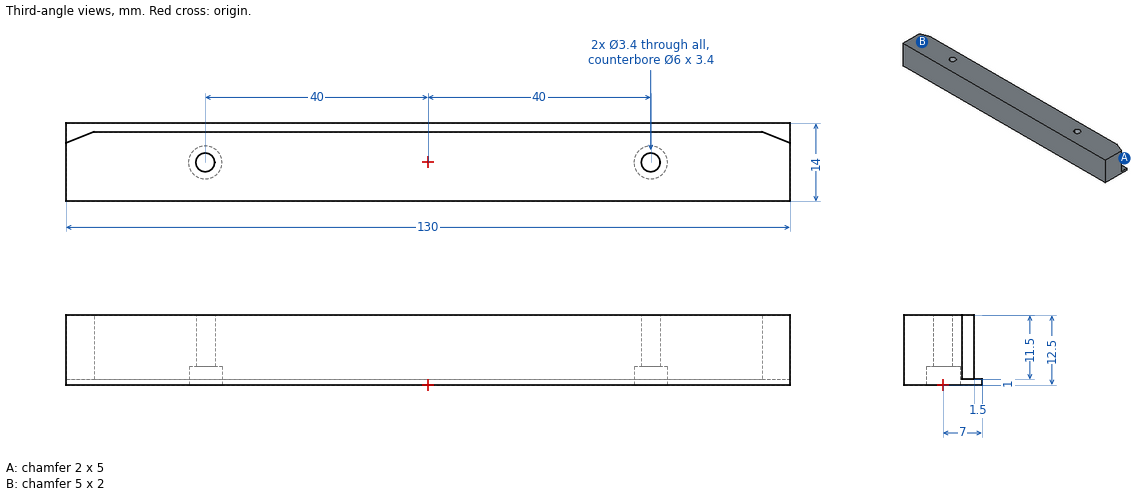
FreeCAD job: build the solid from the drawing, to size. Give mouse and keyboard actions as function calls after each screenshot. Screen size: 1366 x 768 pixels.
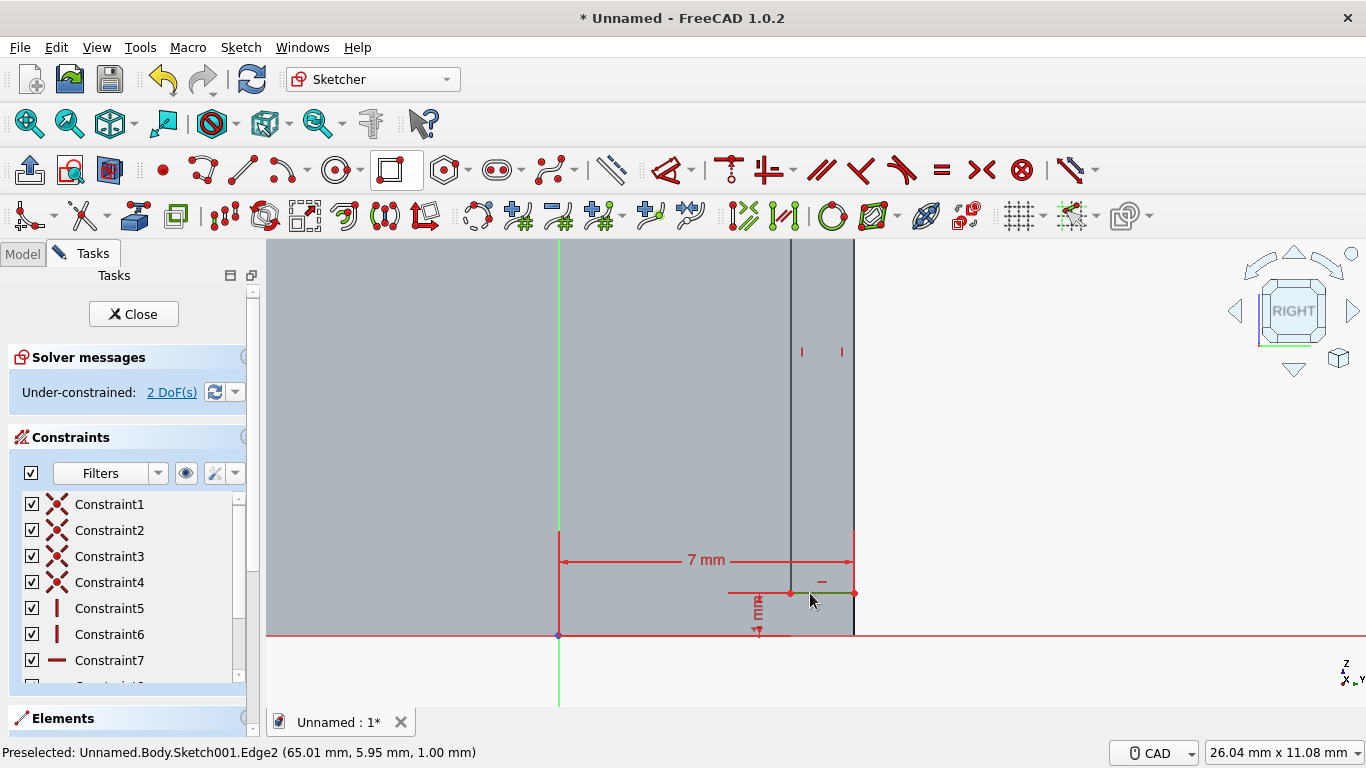
key(l)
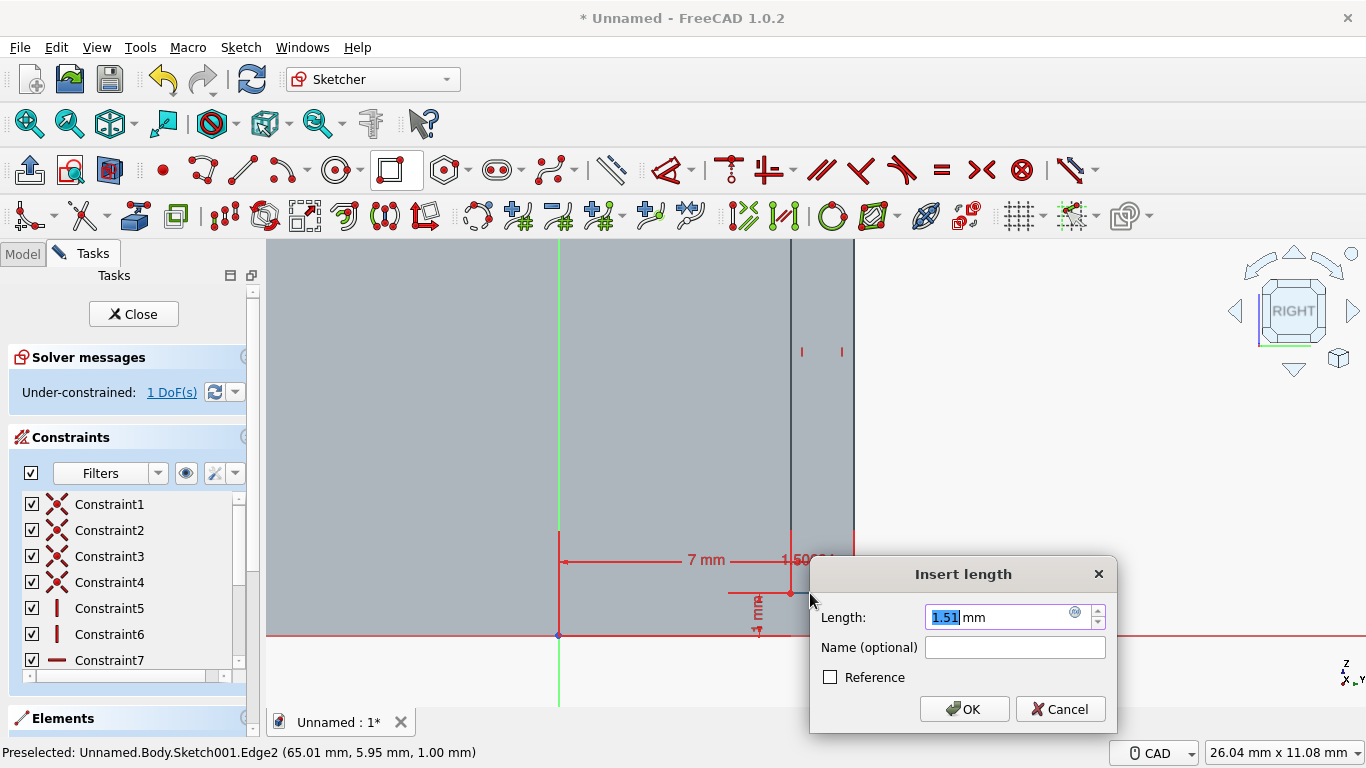
text(1.5)
key(Return)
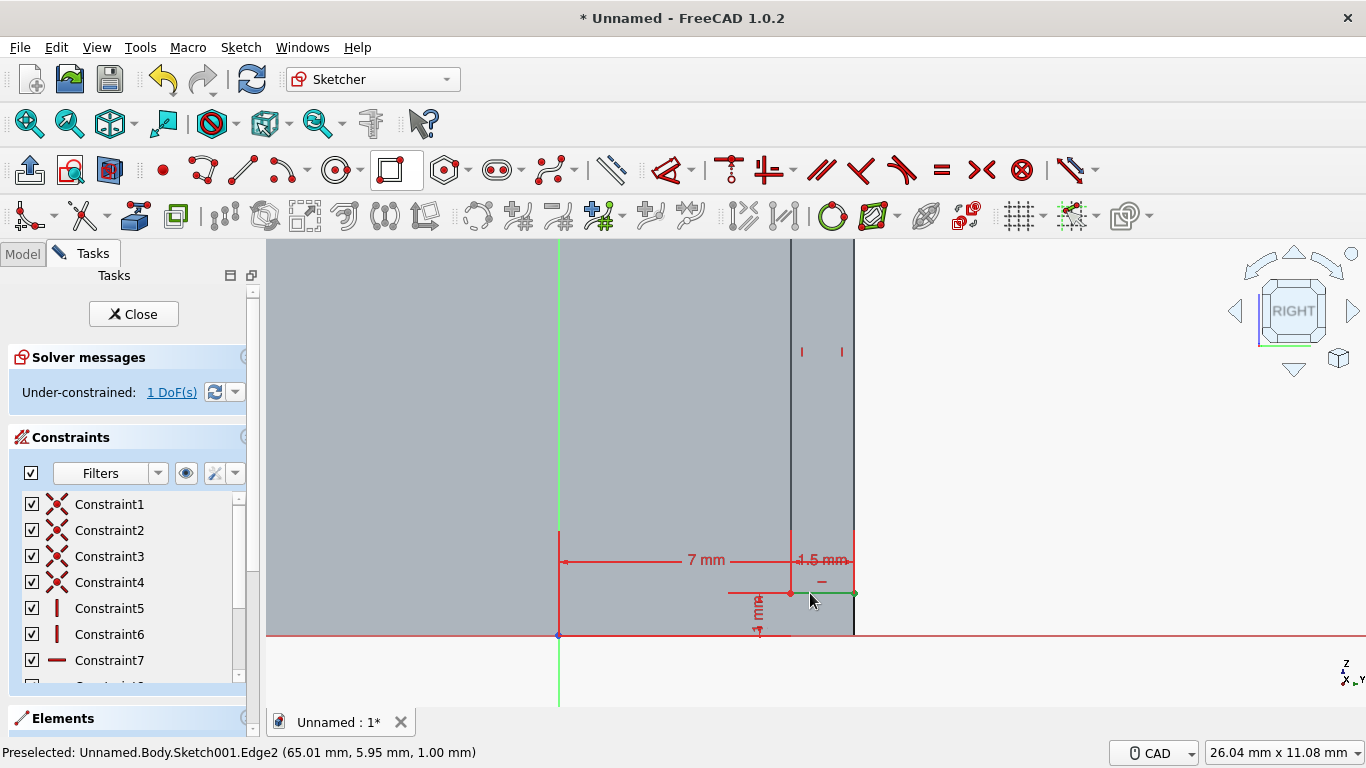
click(791, 448)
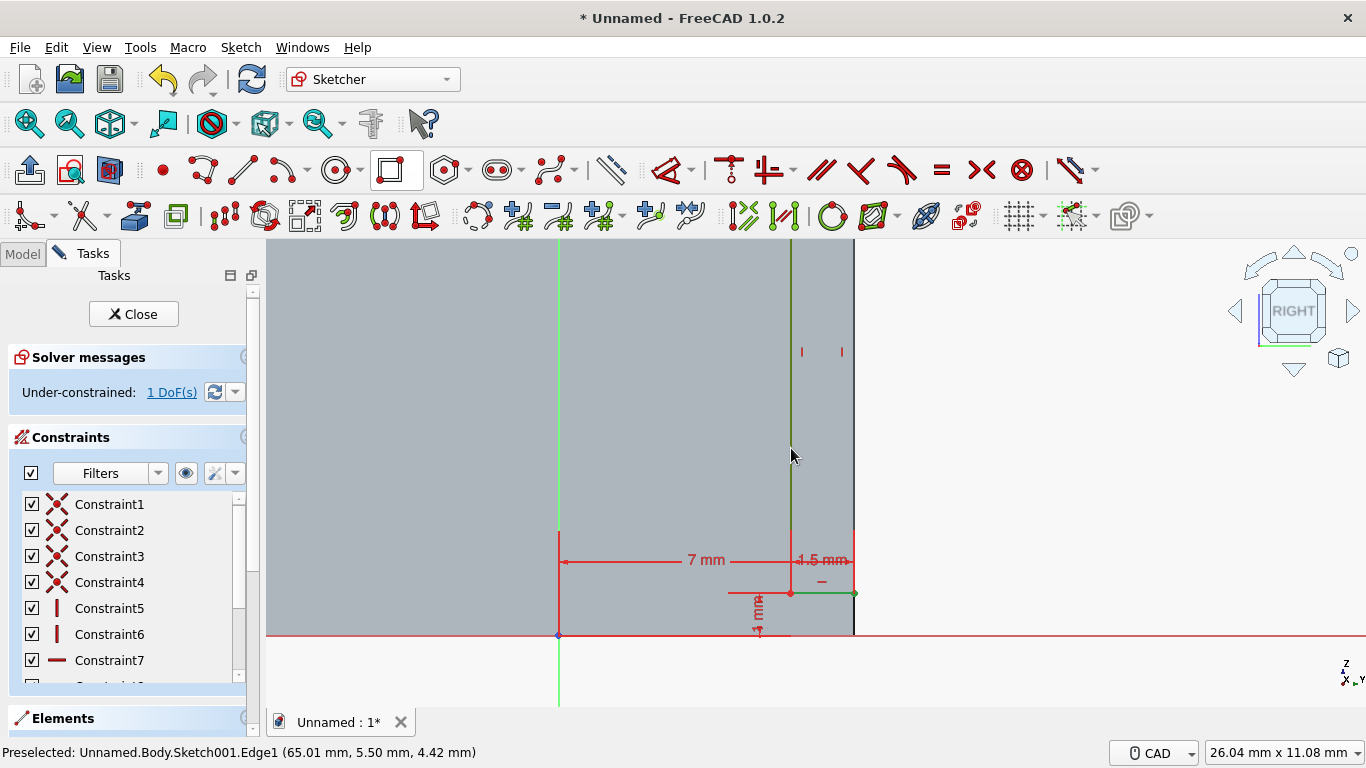
click(694, 170)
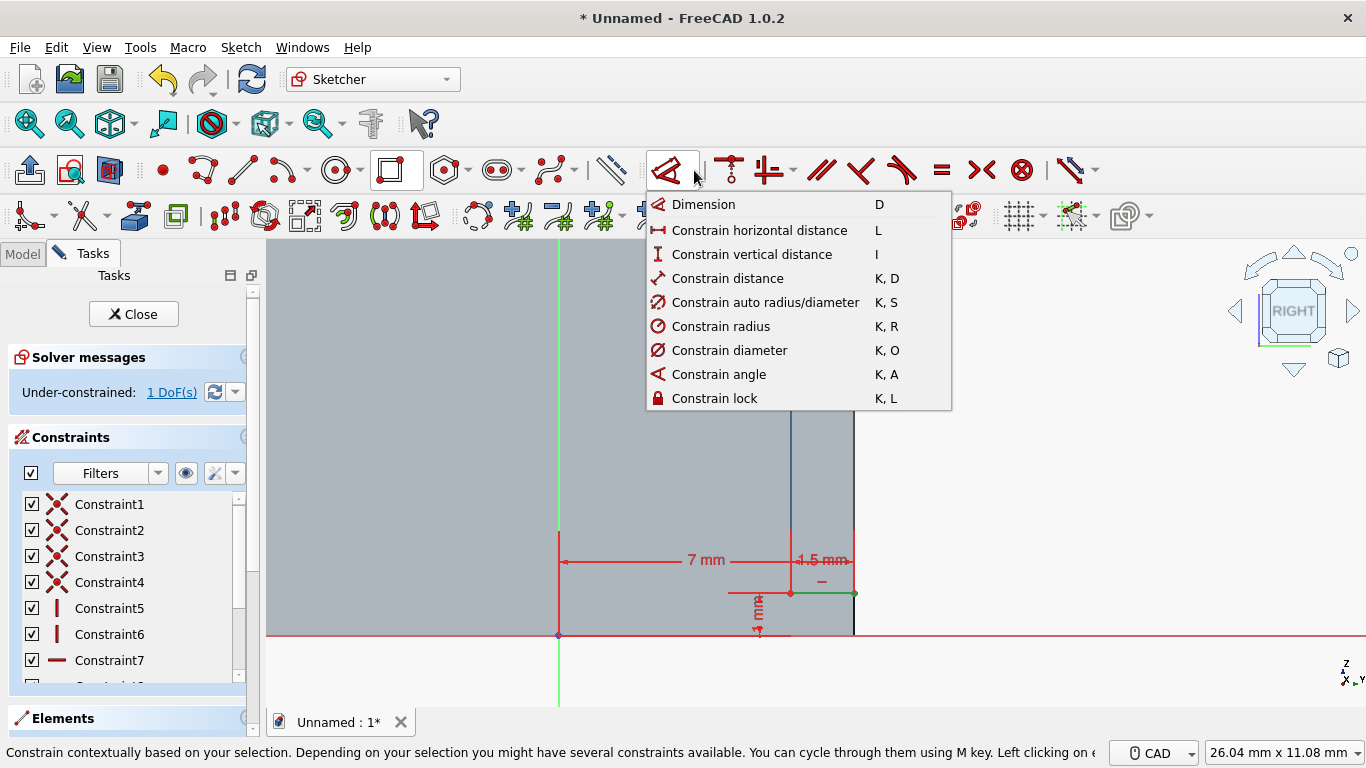
click(799, 254)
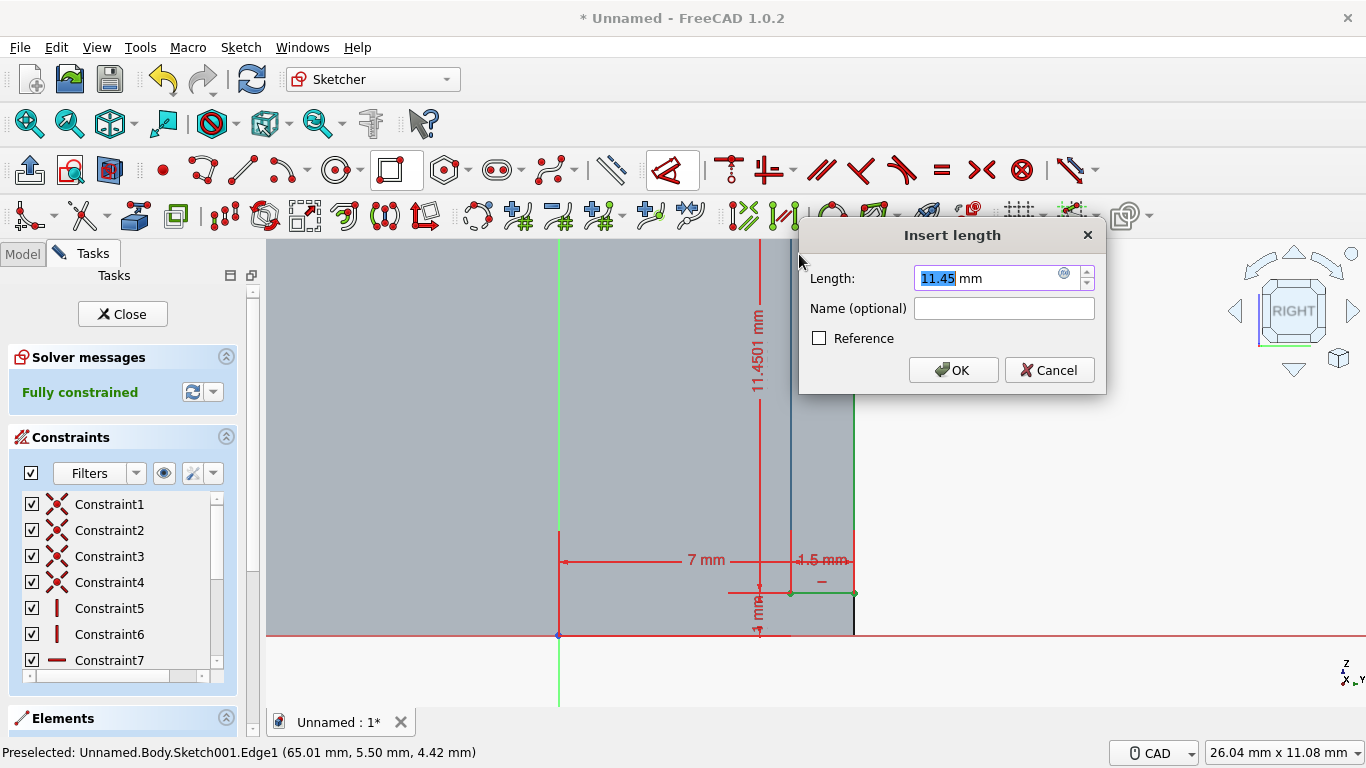
text(11.5)
key(Return)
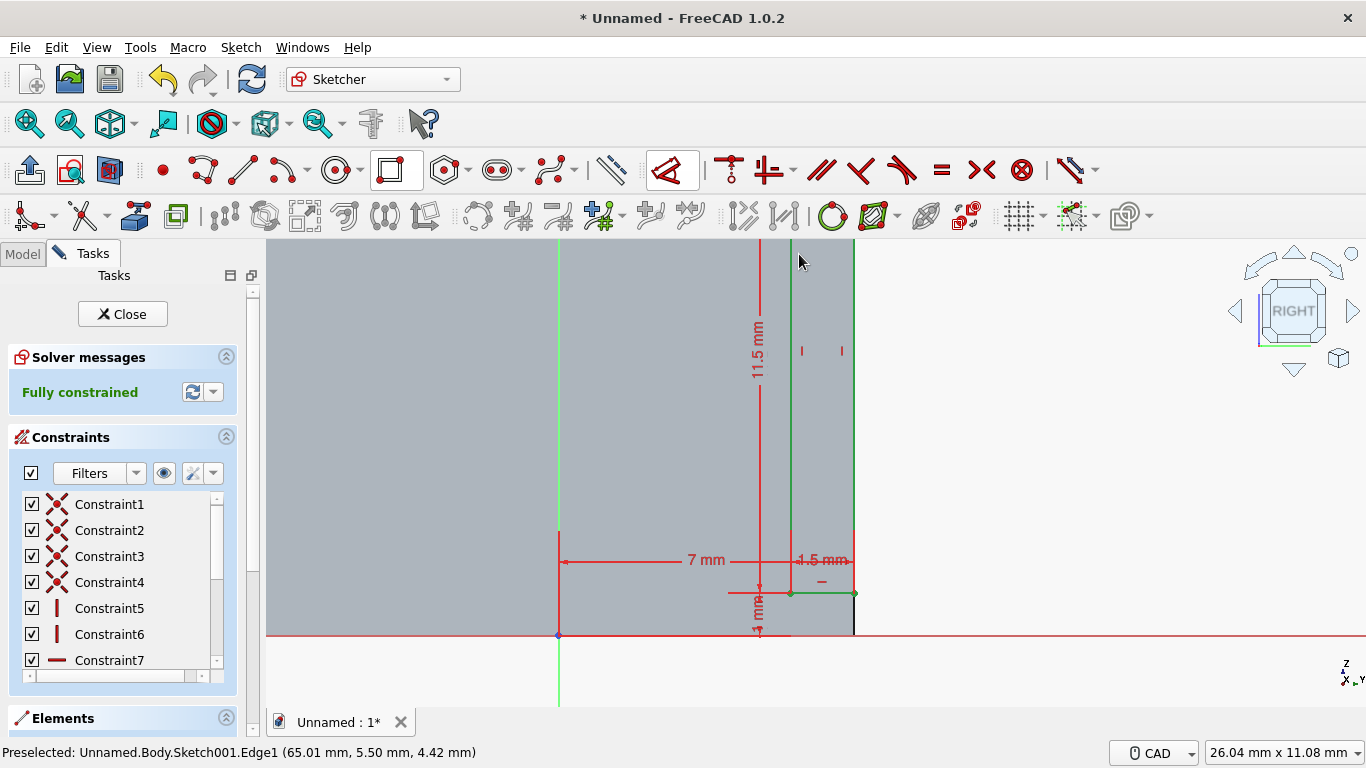
click(123, 314)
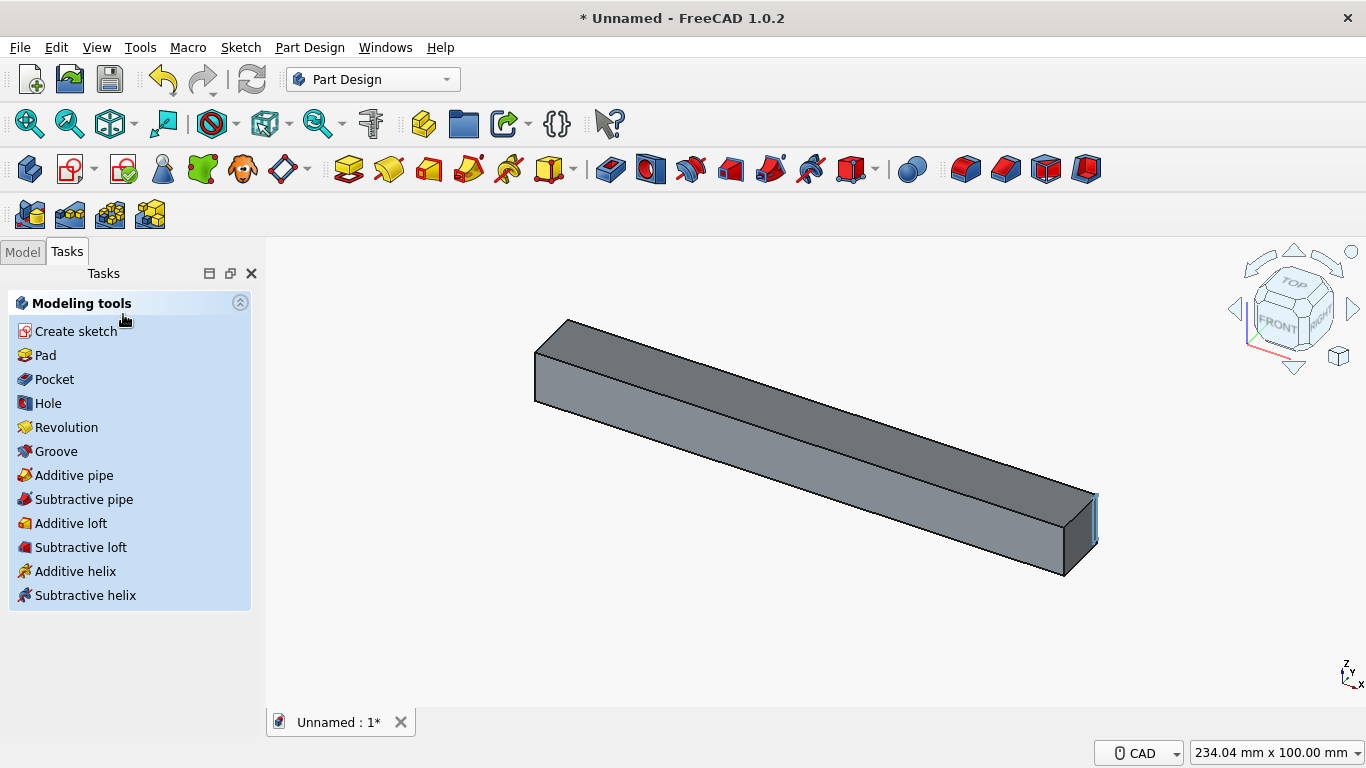
click(612, 170)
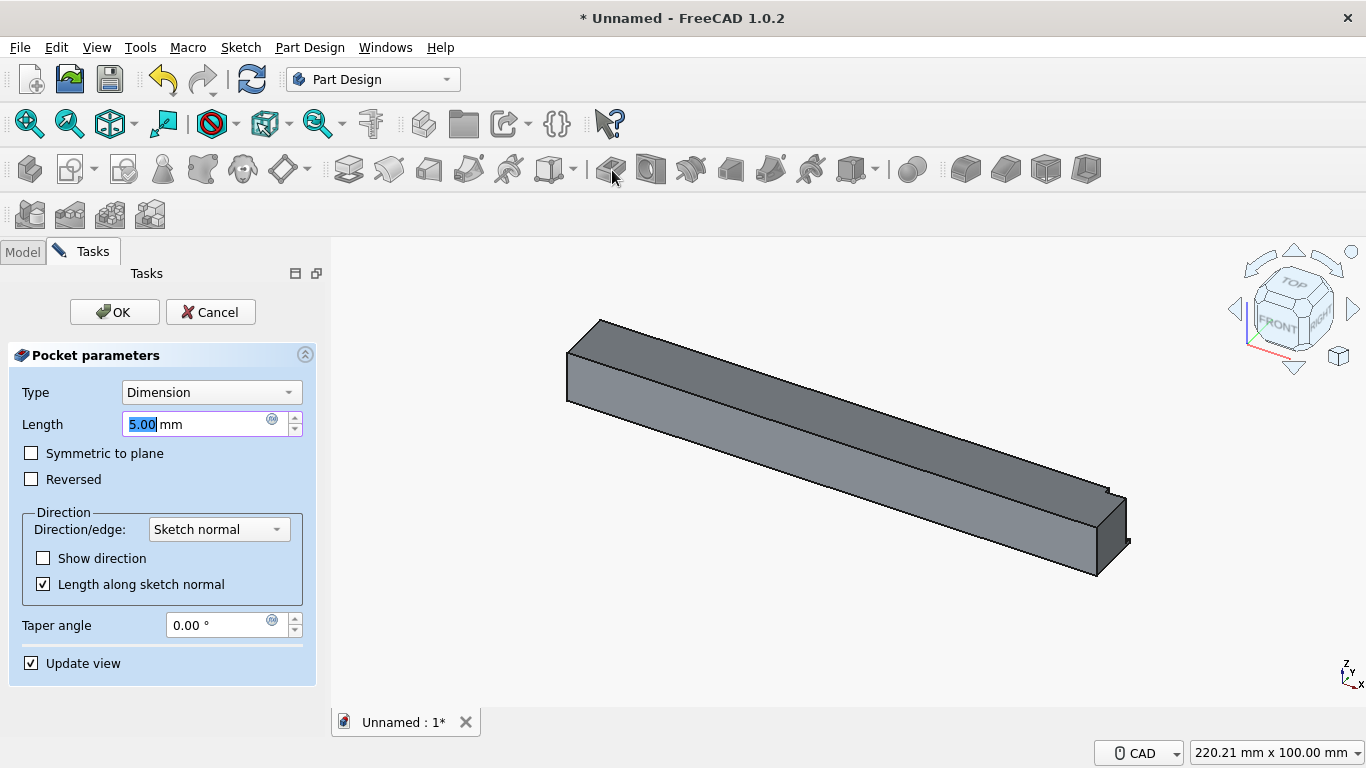
click(212, 392)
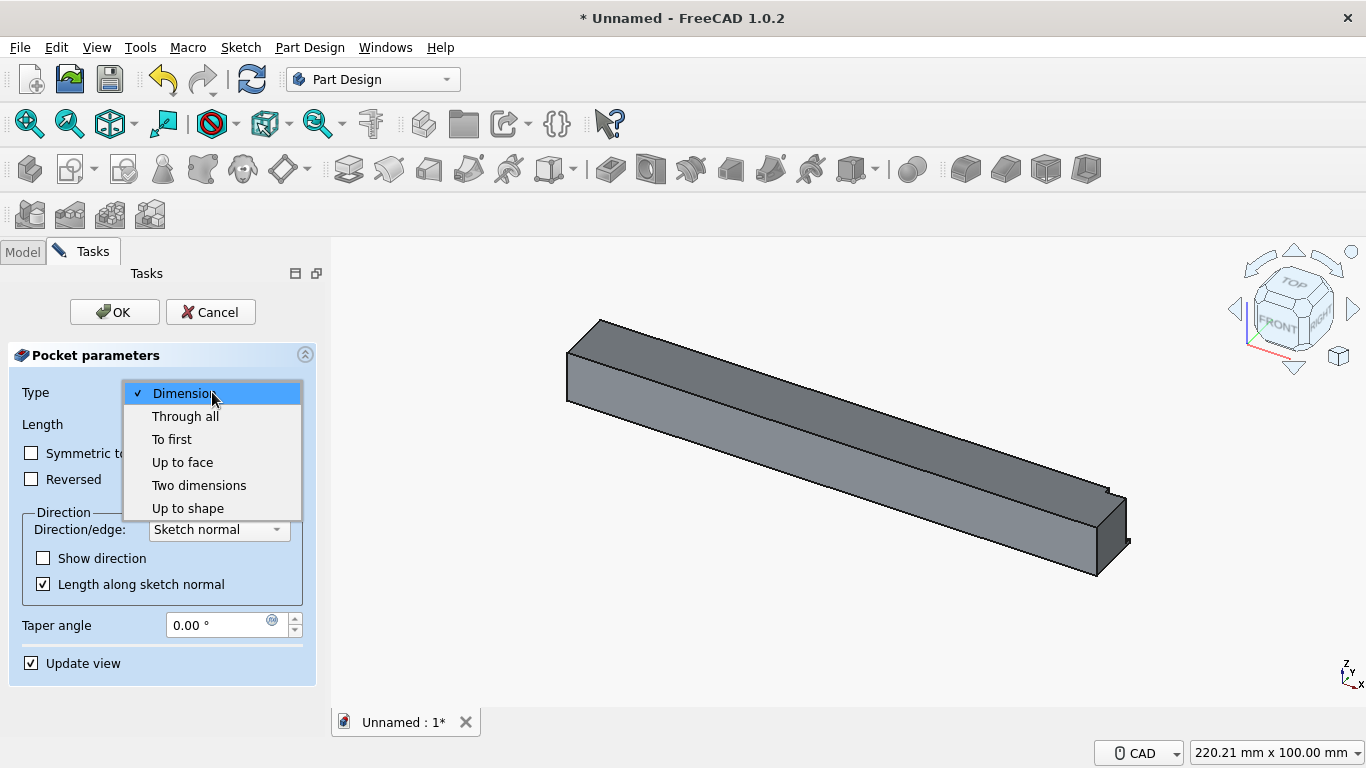
click(212, 416)